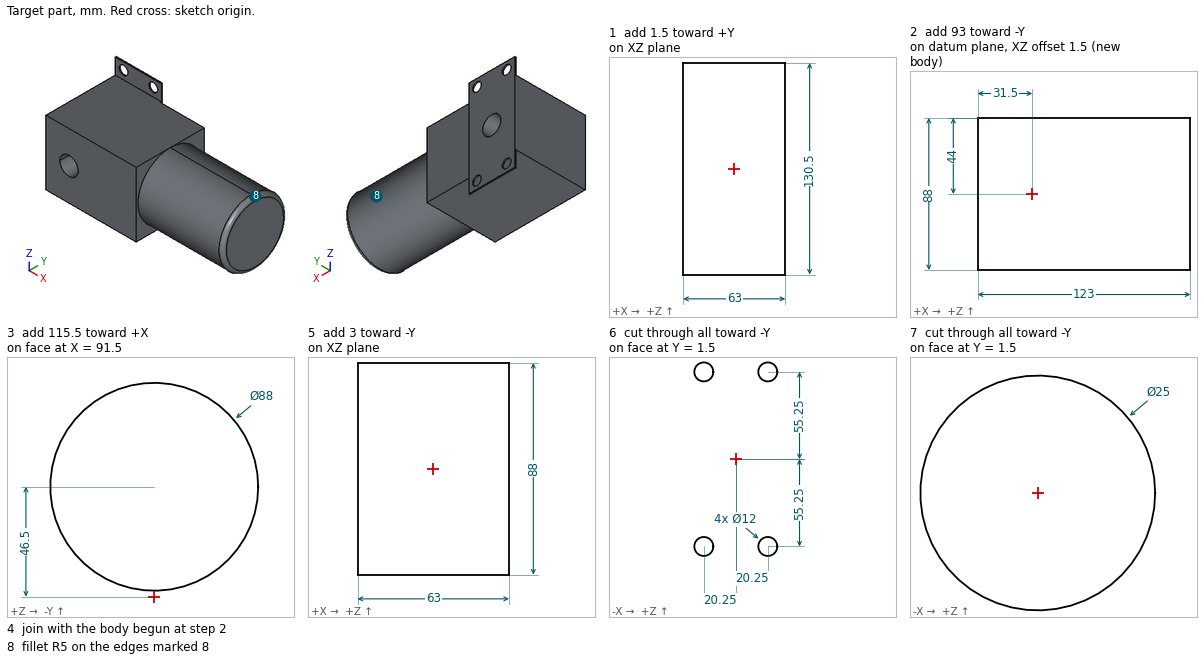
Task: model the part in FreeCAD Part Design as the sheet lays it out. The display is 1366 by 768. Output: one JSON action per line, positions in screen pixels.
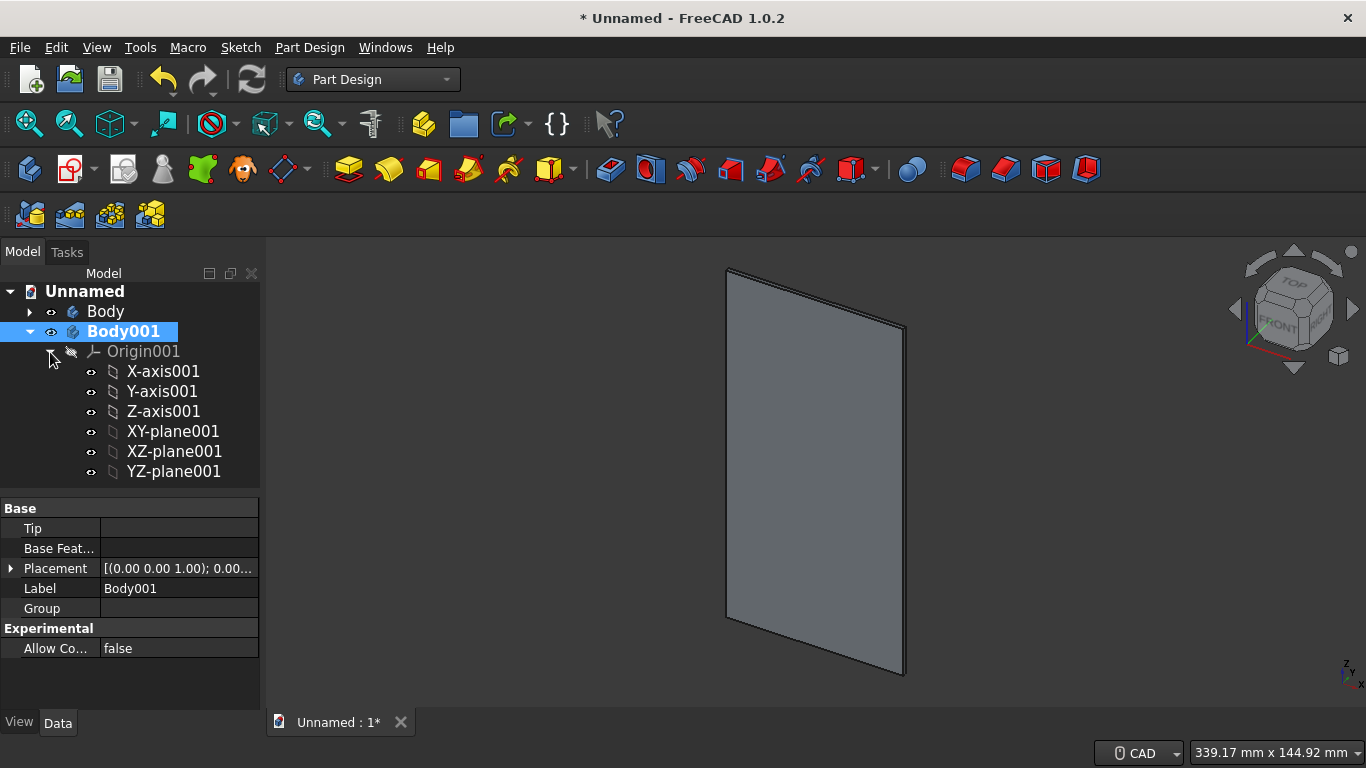
{"action": "left_click", "coordinate": [136, 452]}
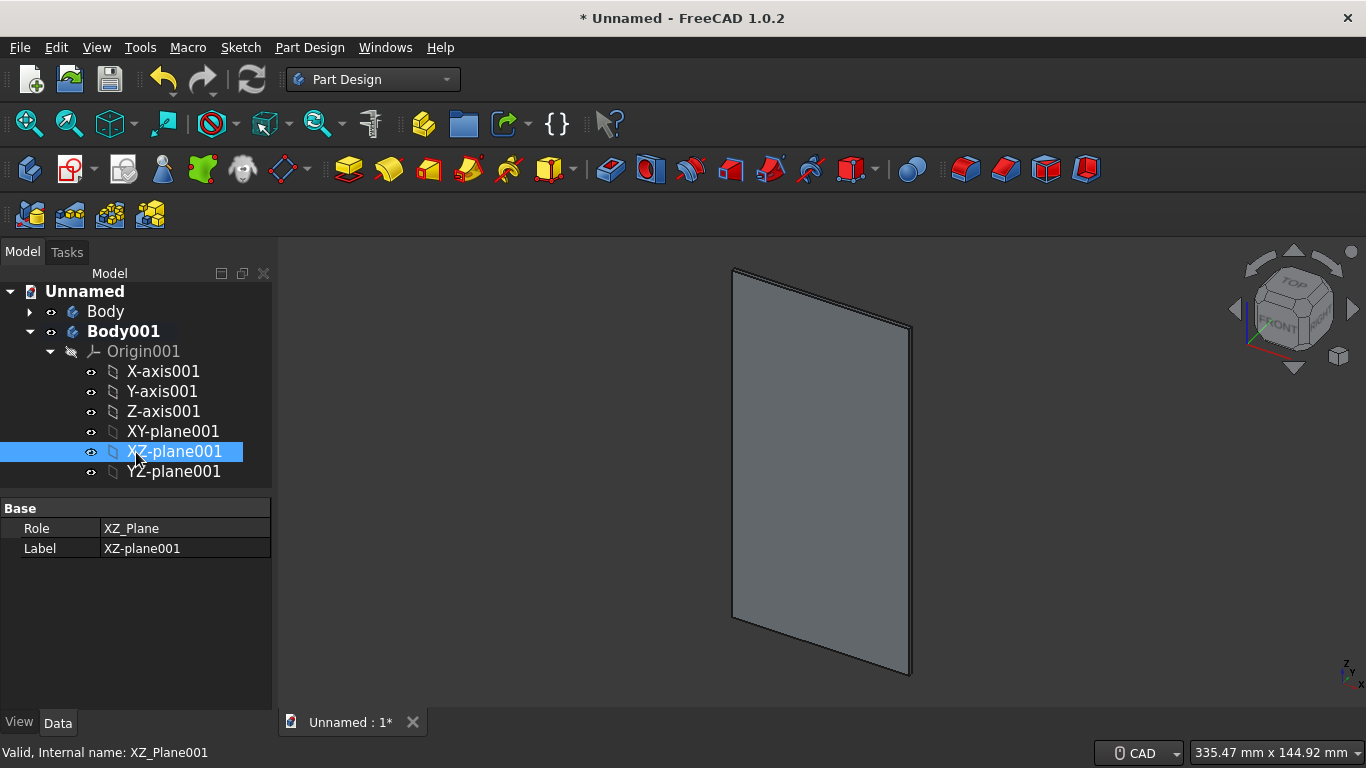
{"action": "left_click", "coordinate": [284, 170]}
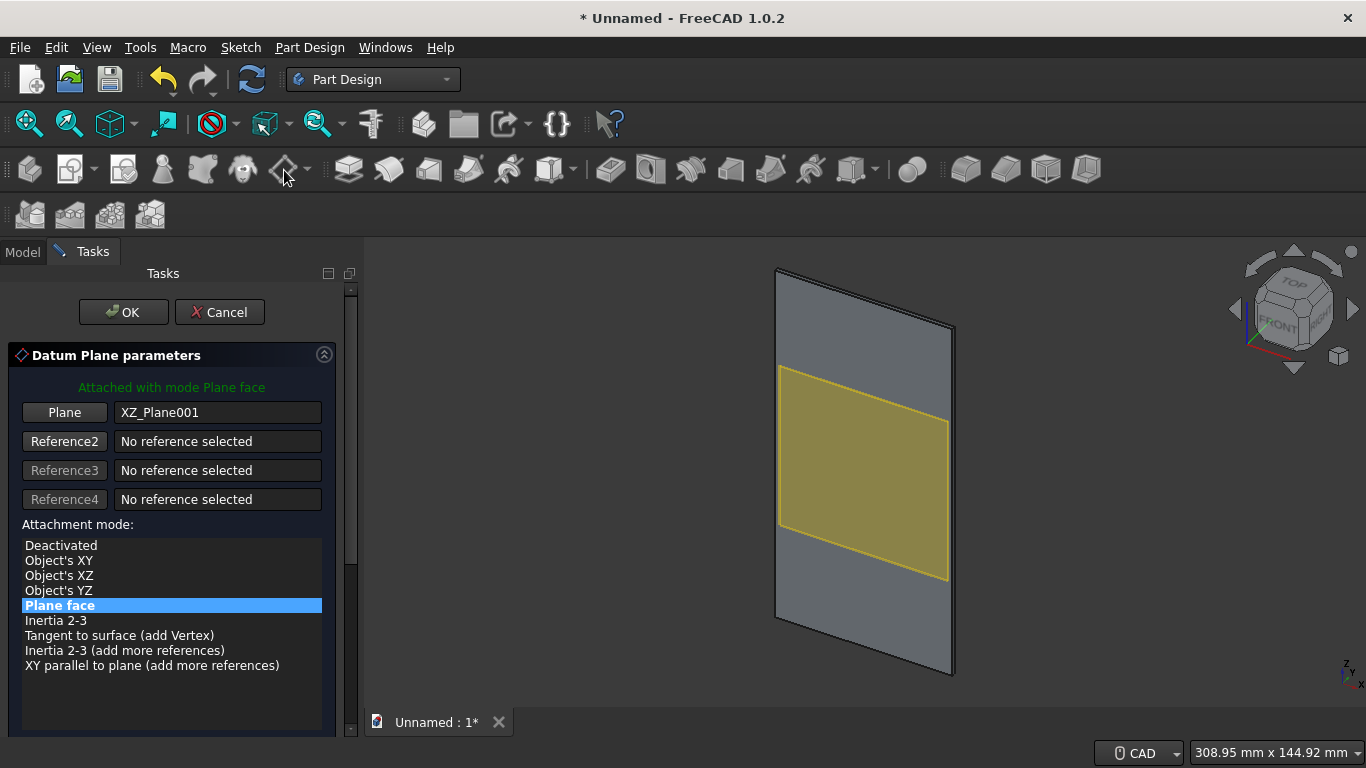
{"action": "scroll", "coordinate": [351, 510], "scroll_direction": "down", "scroll_amount": 3}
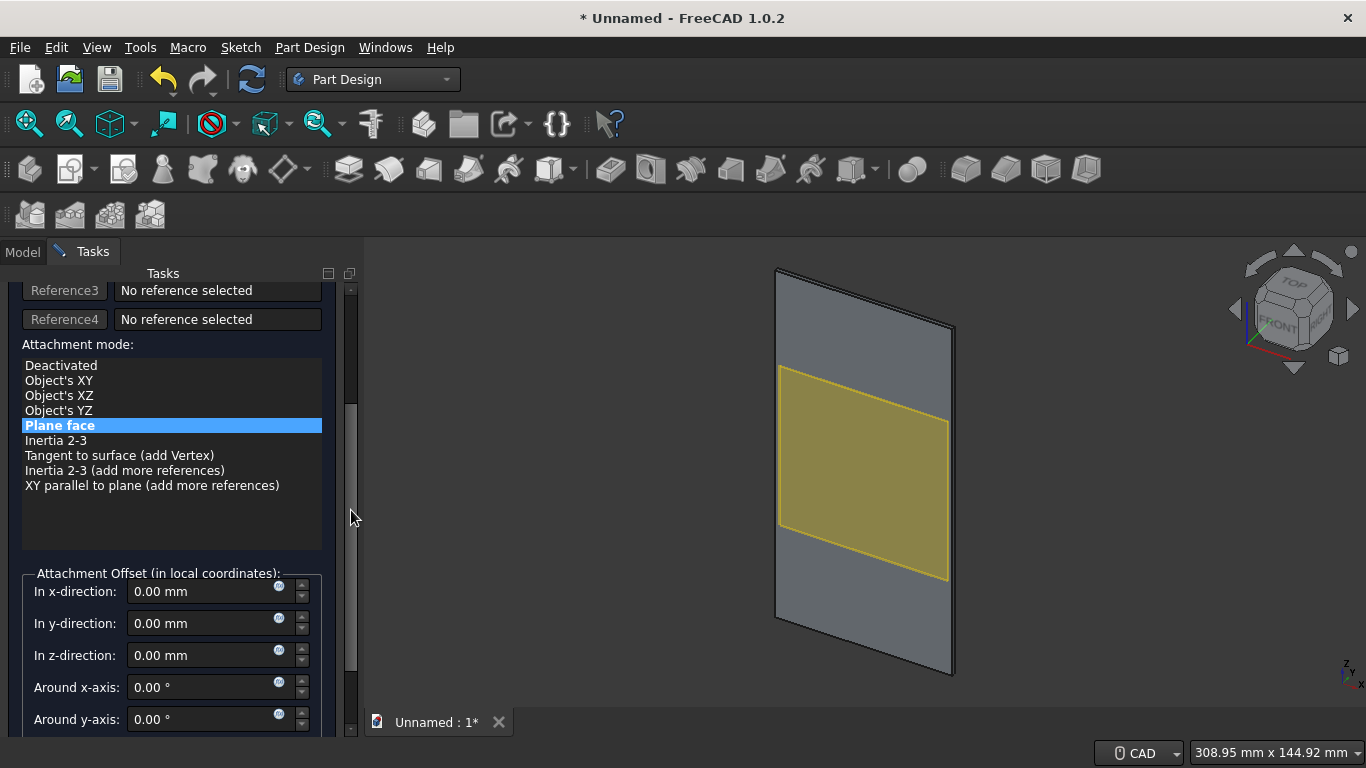
{"action": "triple_click", "coordinate": [210, 655]}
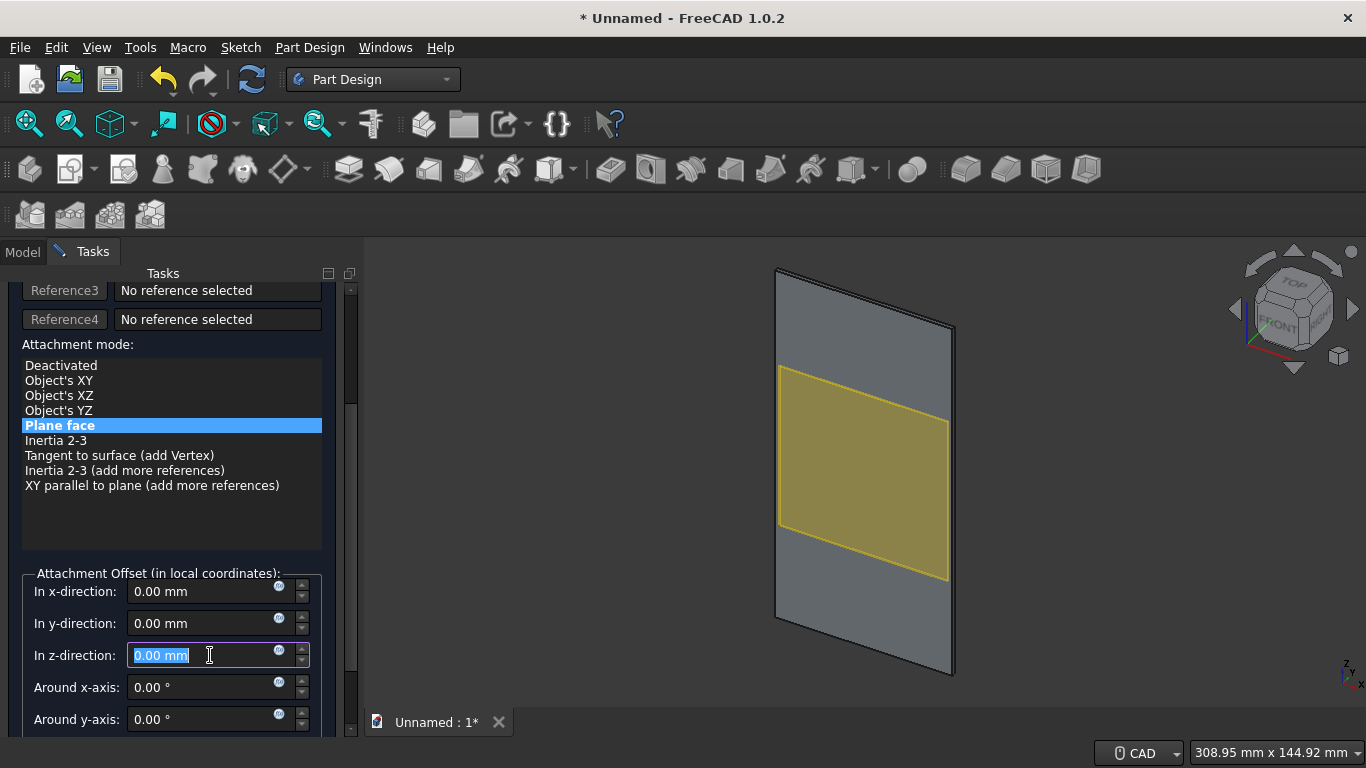
{"action": "type", "text": "1.5"}
{"action": "key", "text": "Tab"}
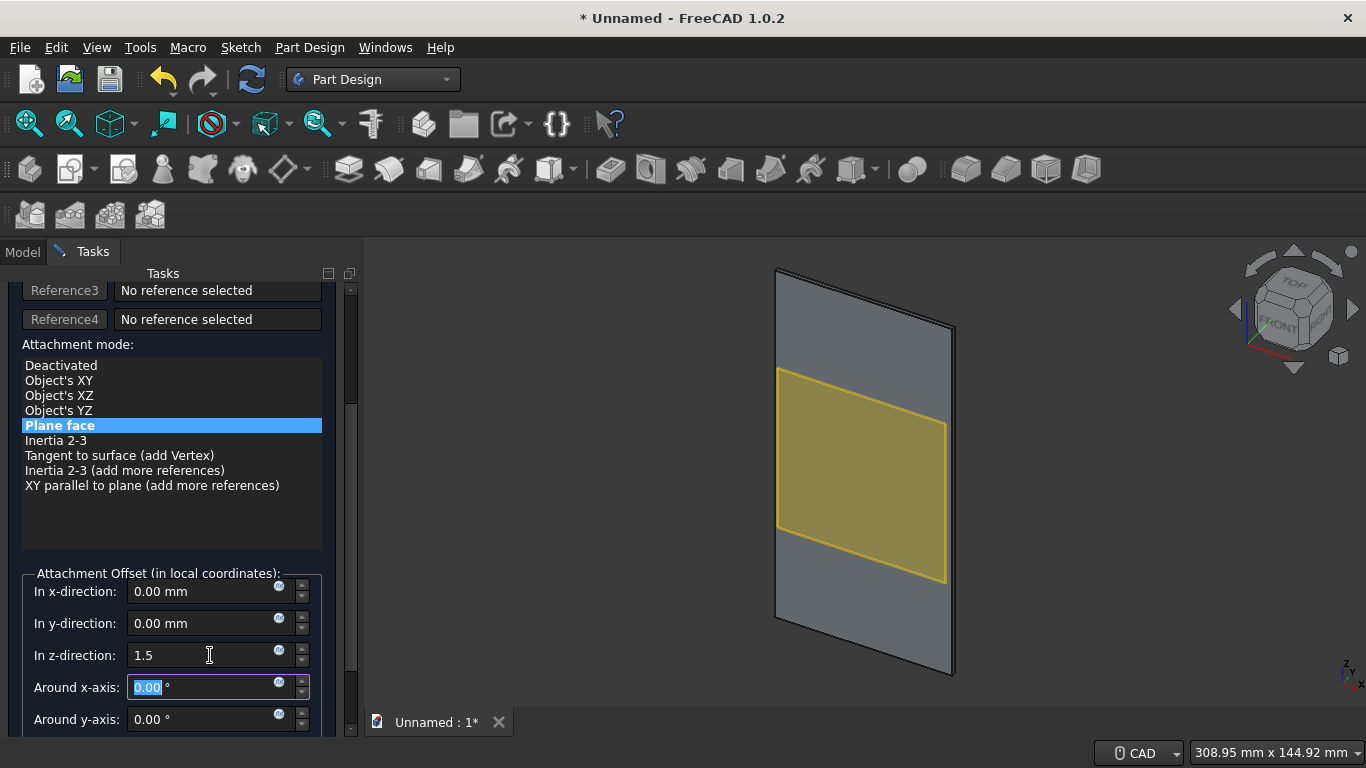
{"action": "scroll", "coordinate": [351, 510], "scroll_direction": "up", "scroll_amount": 4}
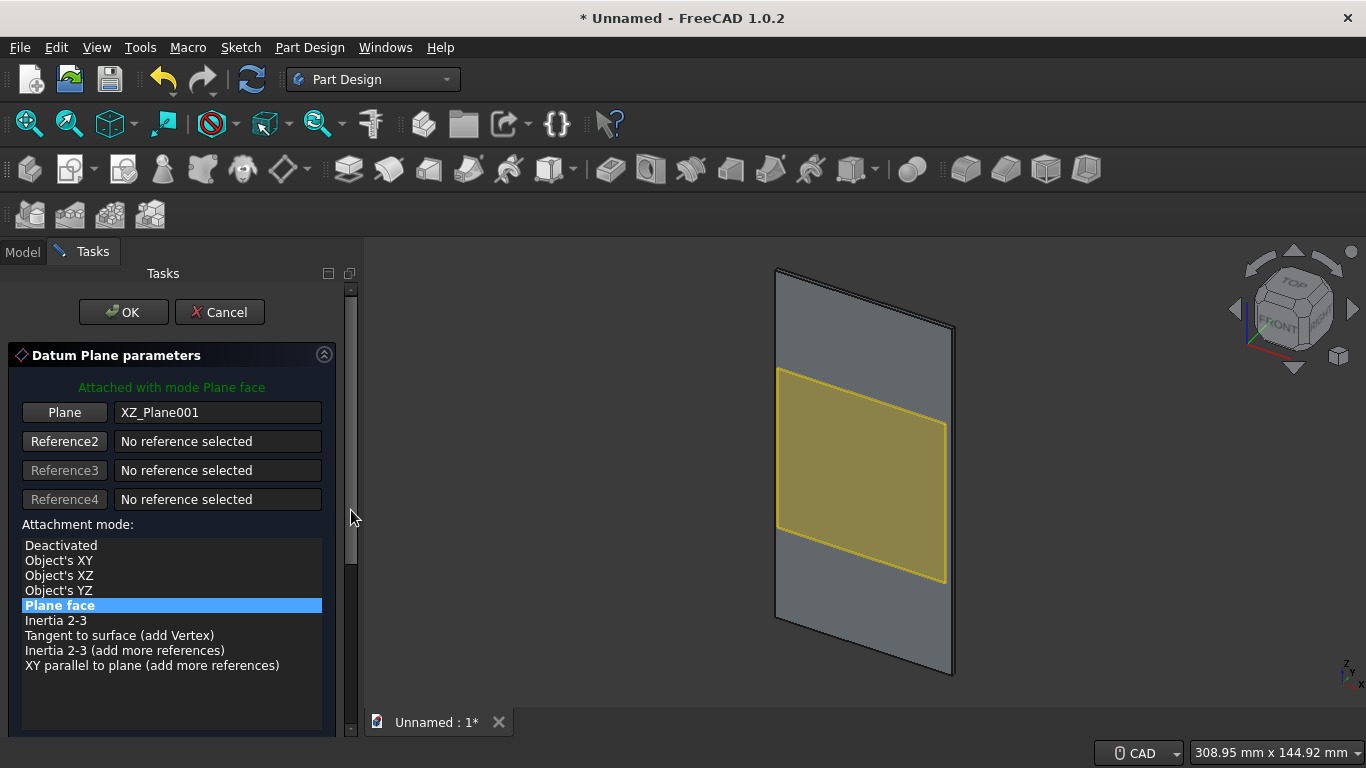
{"action": "left_click", "coordinate": [124, 312]}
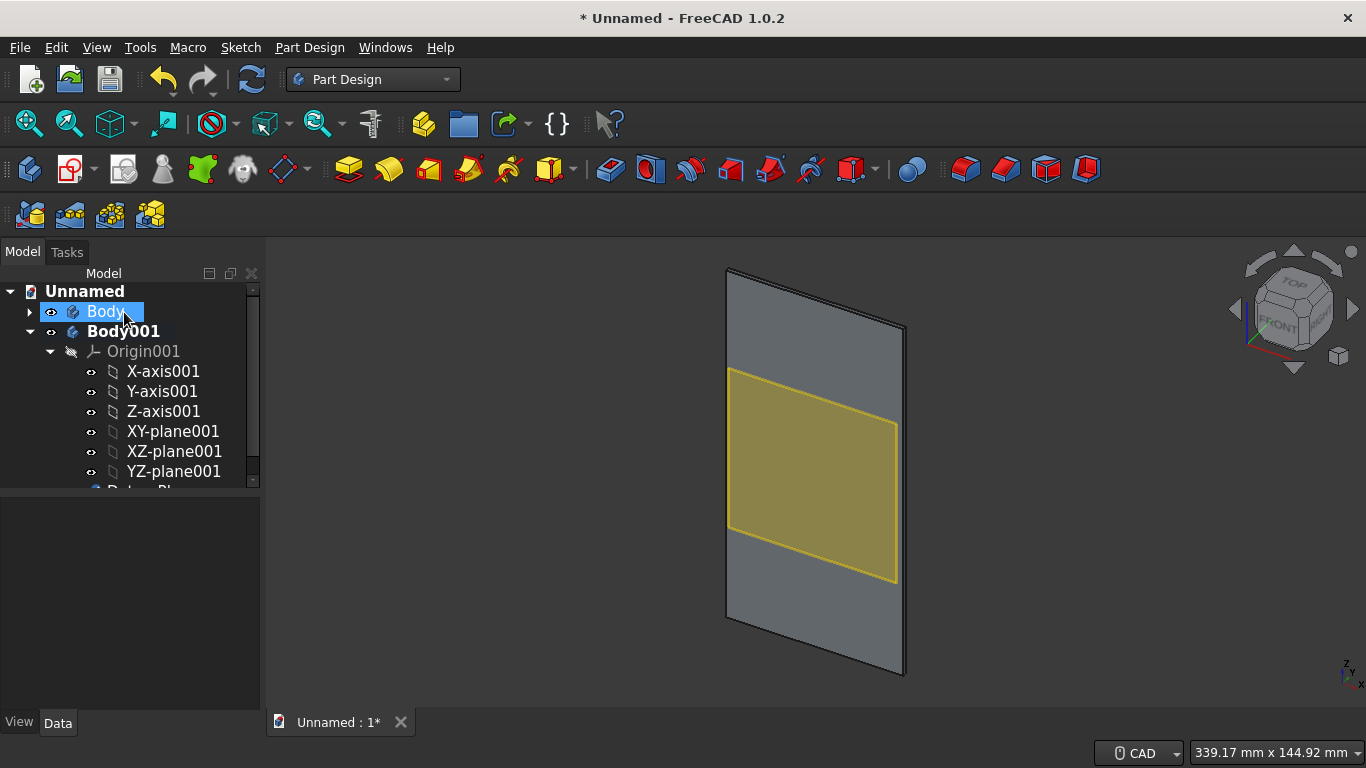
{"action": "scroll", "coordinate": [100, 387], "scroll_direction": "down", "scroll_amount": 3}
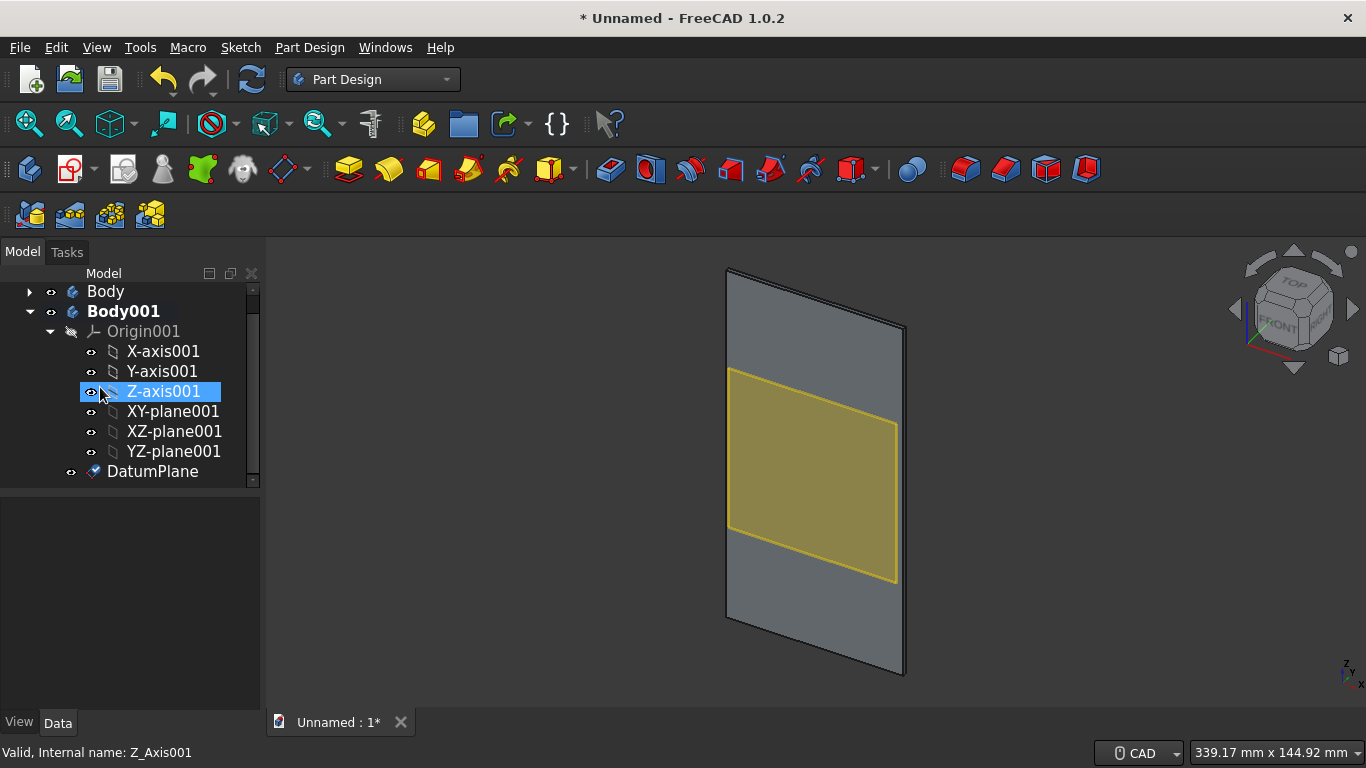
{"action": "left_click", "coordinate": [116, 472]}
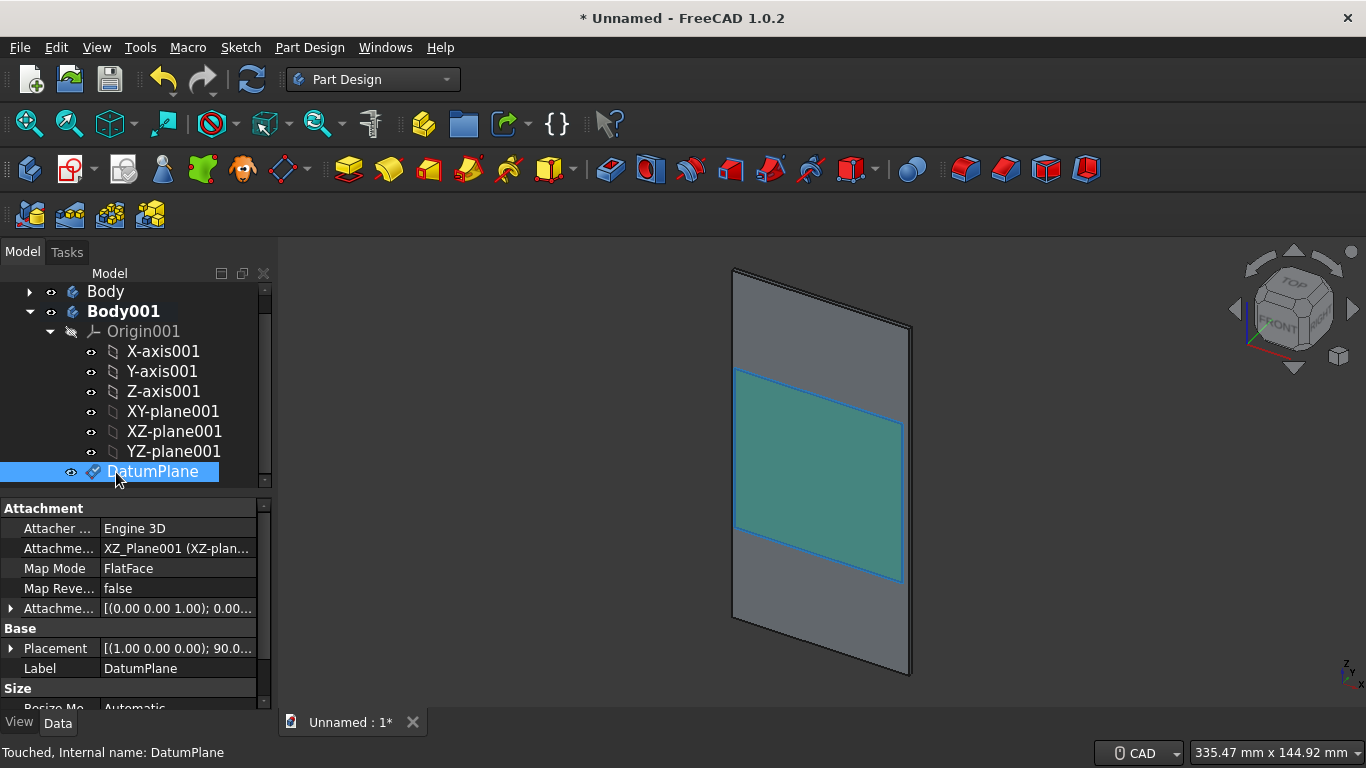
{"action": "left_click", "coordinate": [70, 170]}